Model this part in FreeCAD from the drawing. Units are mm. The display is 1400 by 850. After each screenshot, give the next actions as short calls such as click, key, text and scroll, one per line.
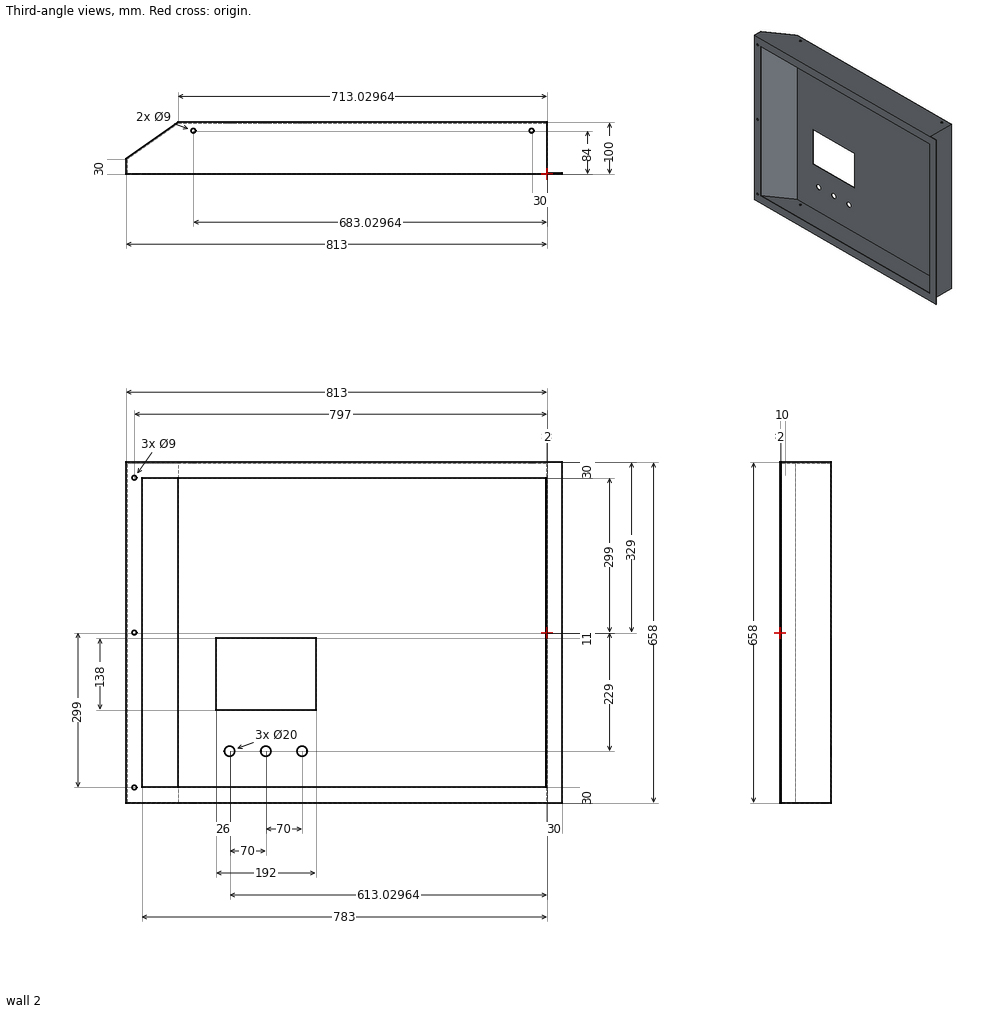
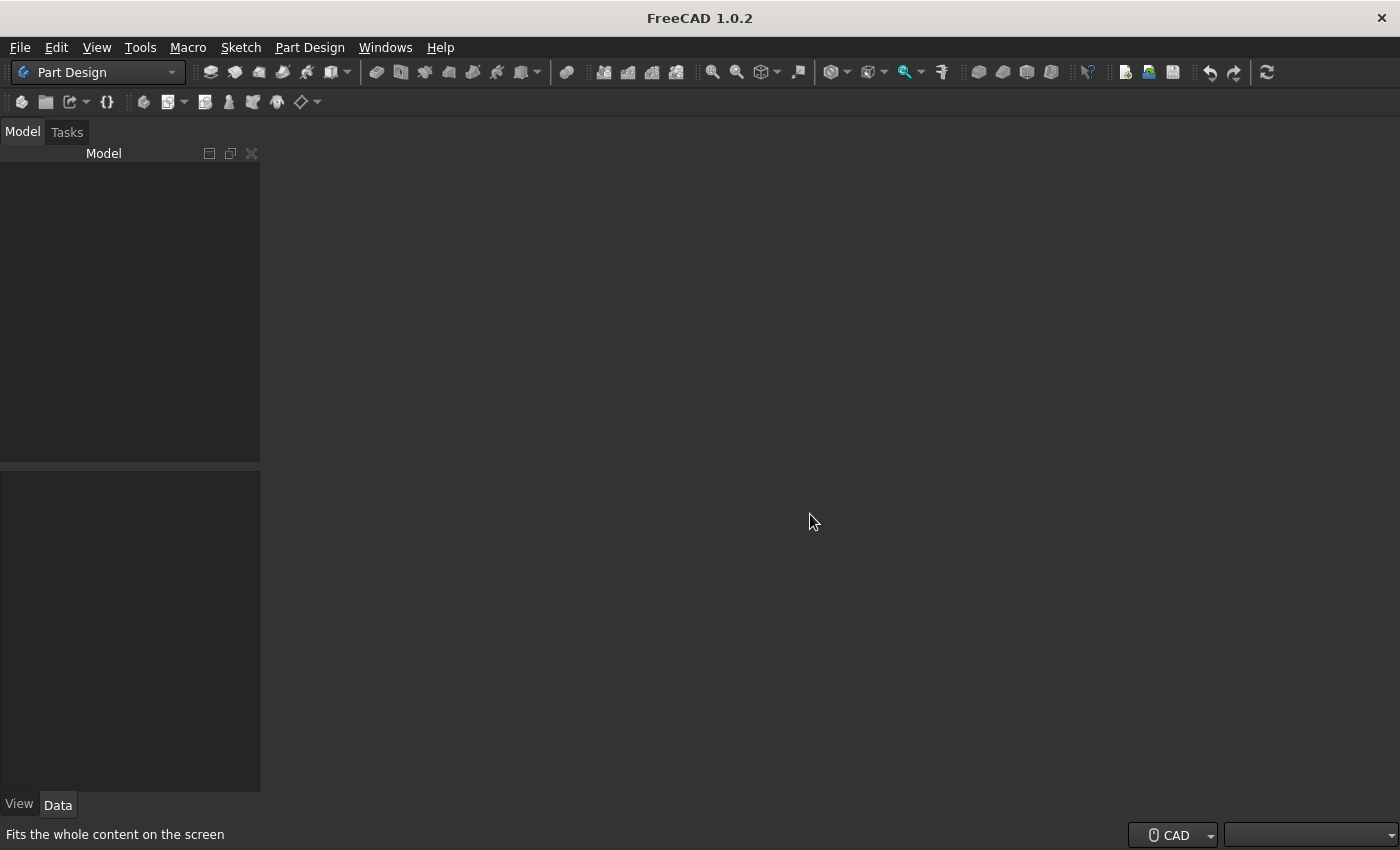
click(1126, 72)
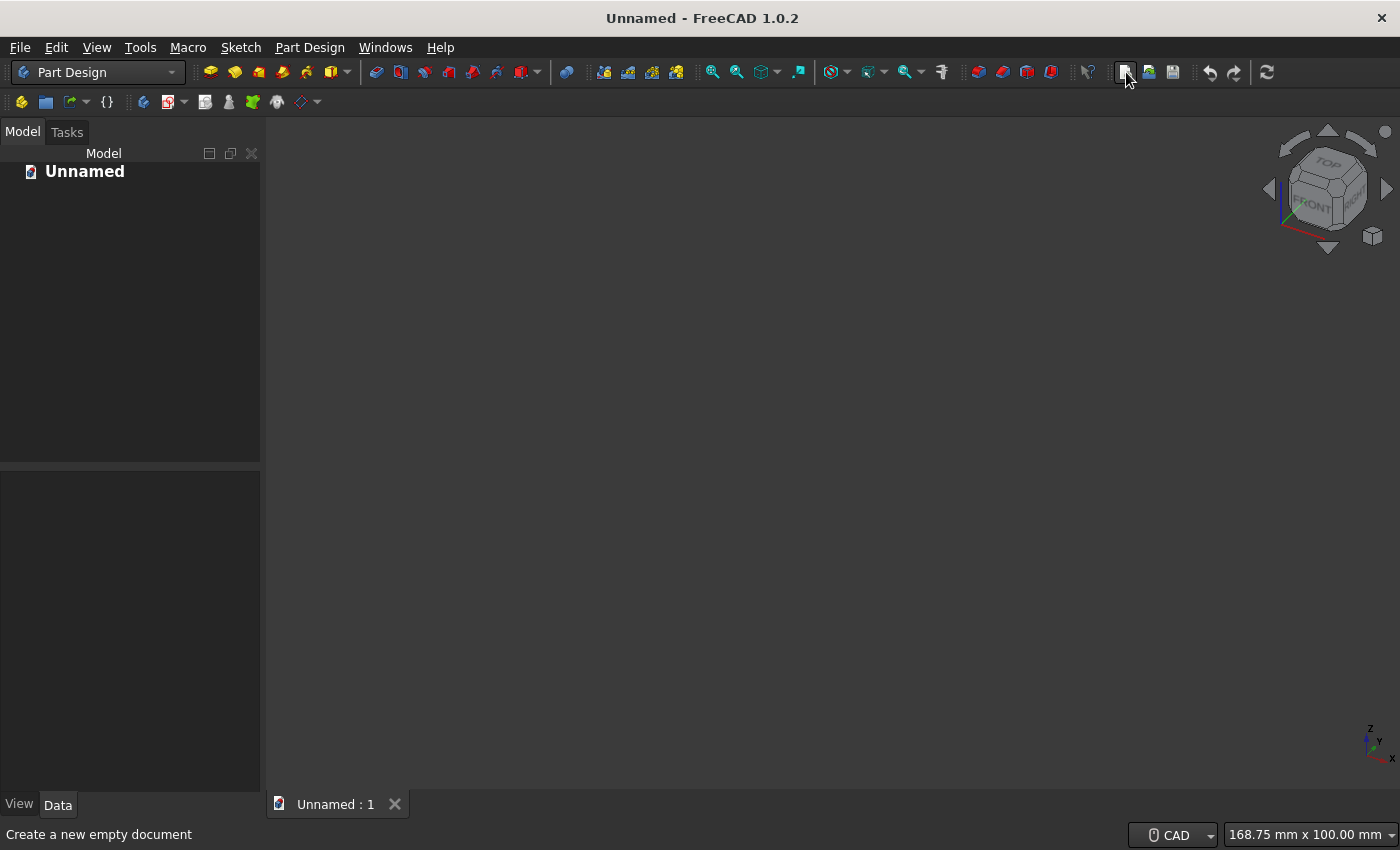
click(168, 102)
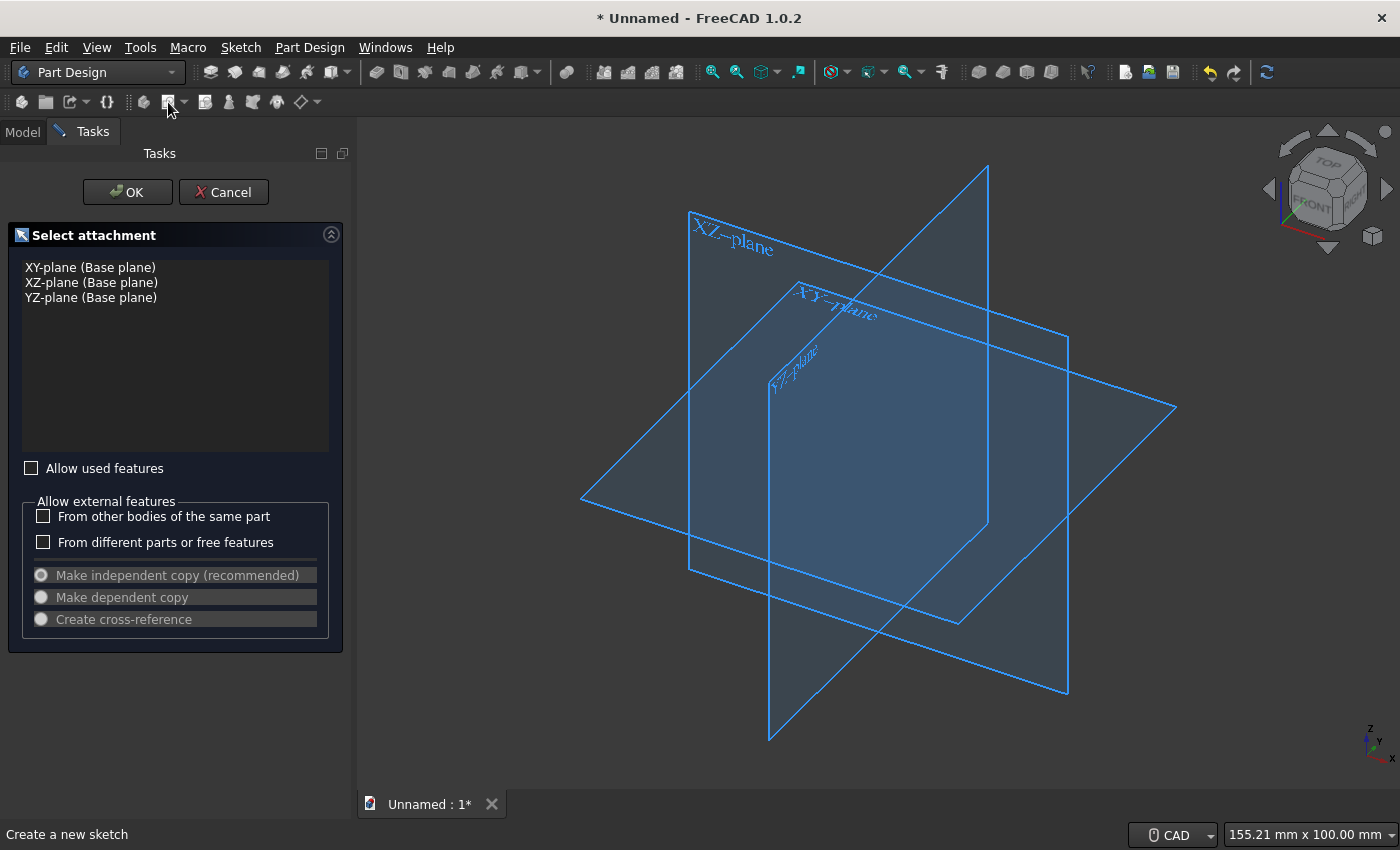
click(82, 268)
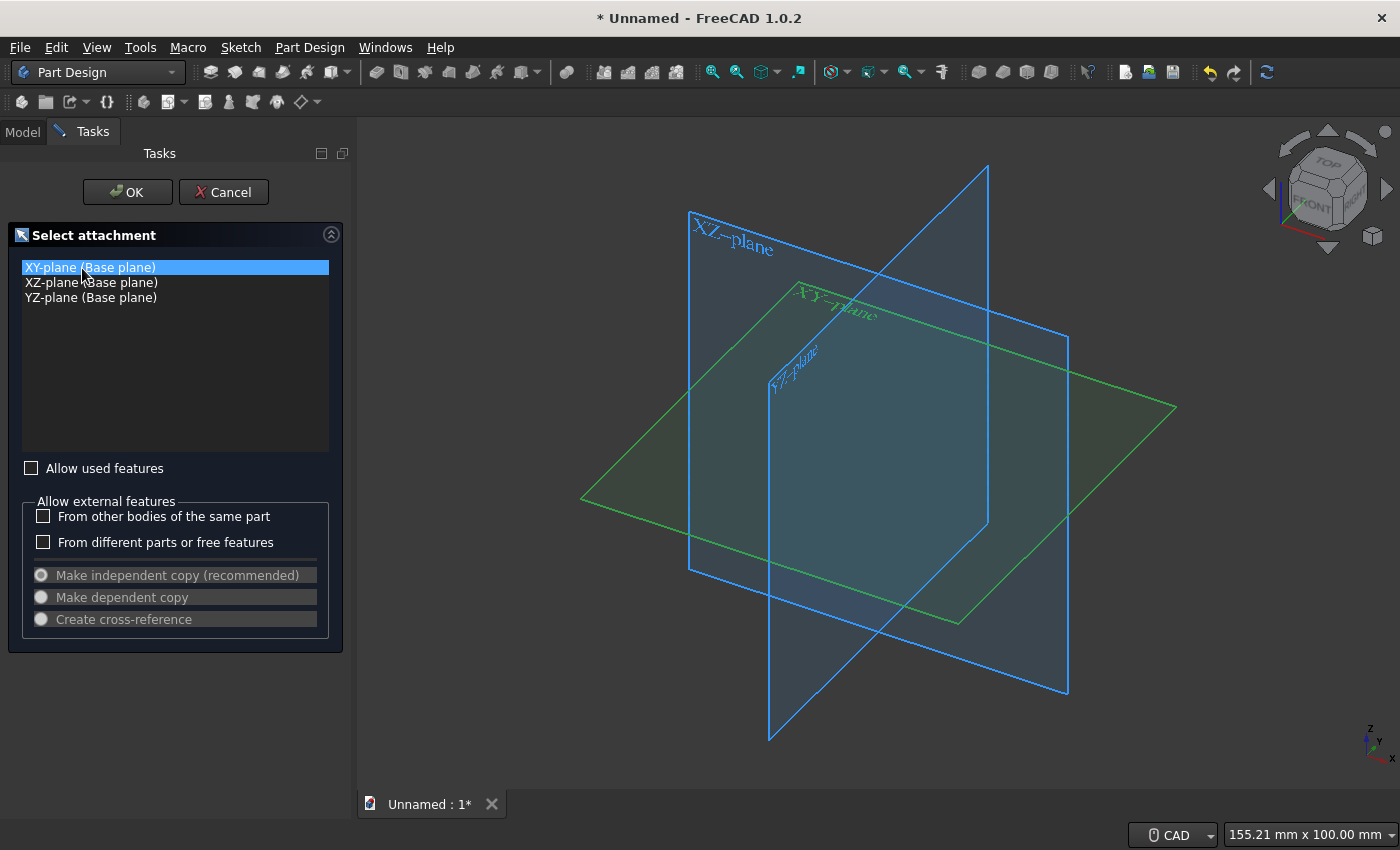
click(128, 192)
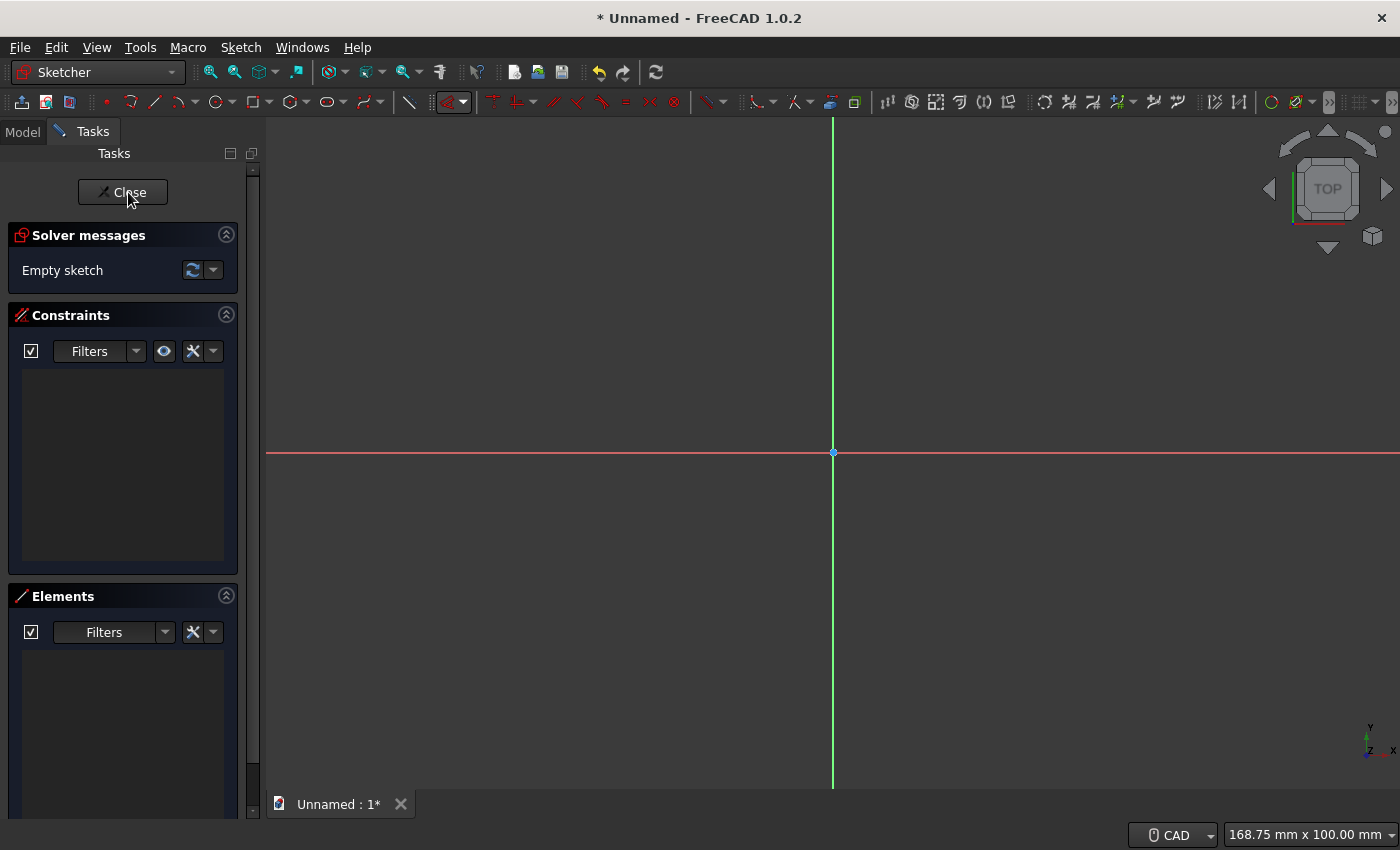
scroll(1096, 495, down, 11)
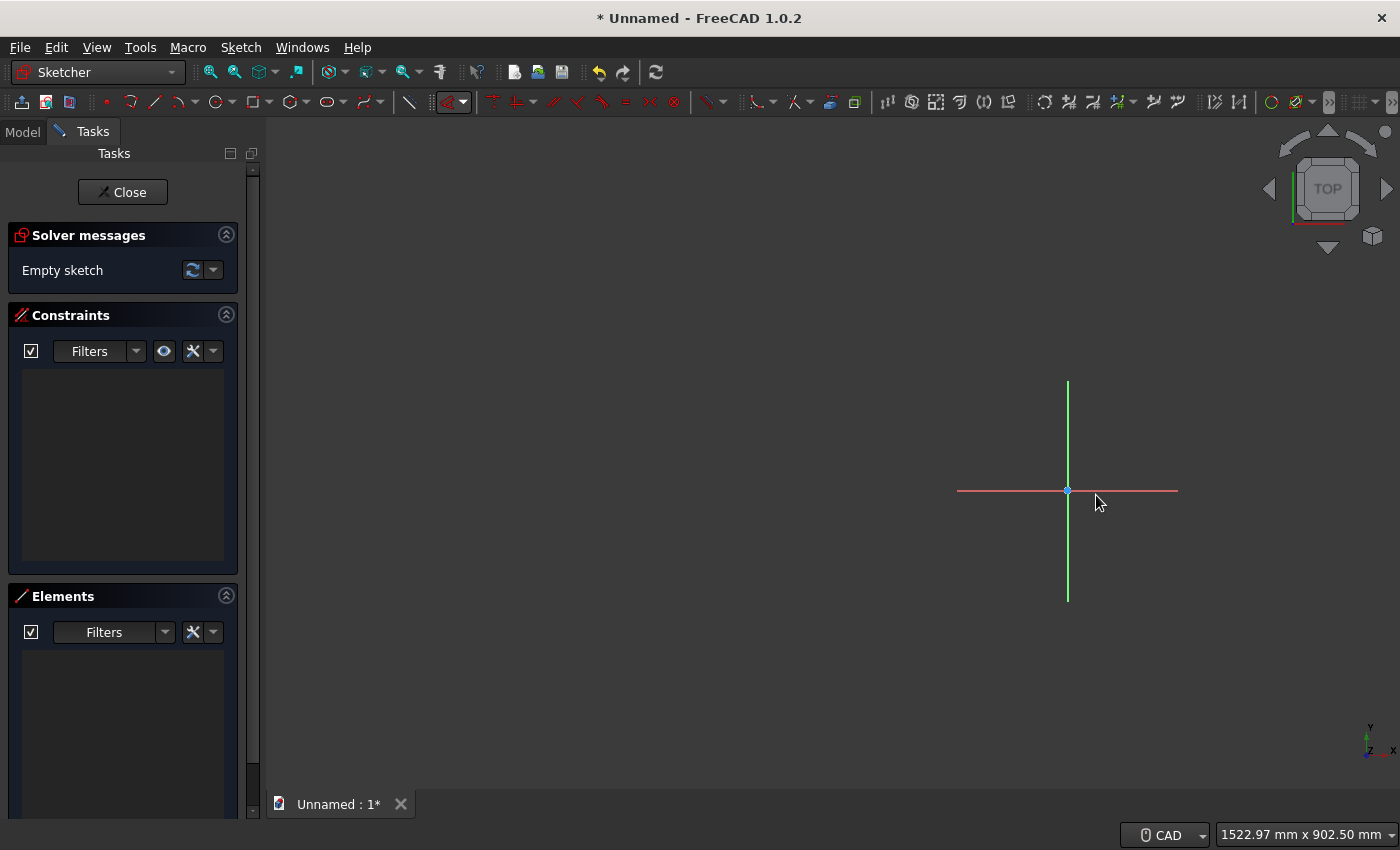
click(132, 102)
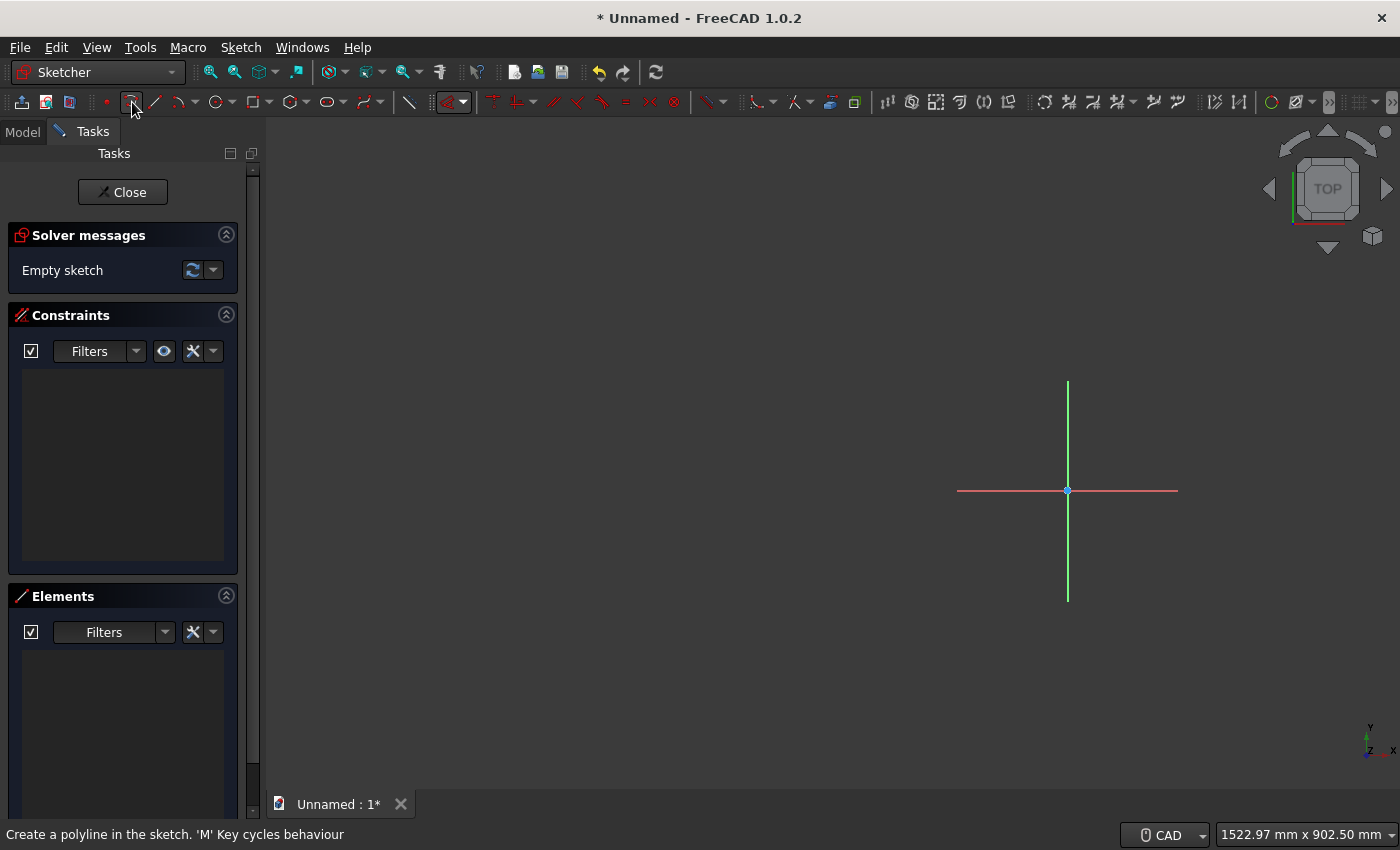
click(1068, 491)
click(1059, 416)
click(537, 416)
click(462, 469)
click(462, 482)
click(1068, 491)
key(Escape)
key(Escape)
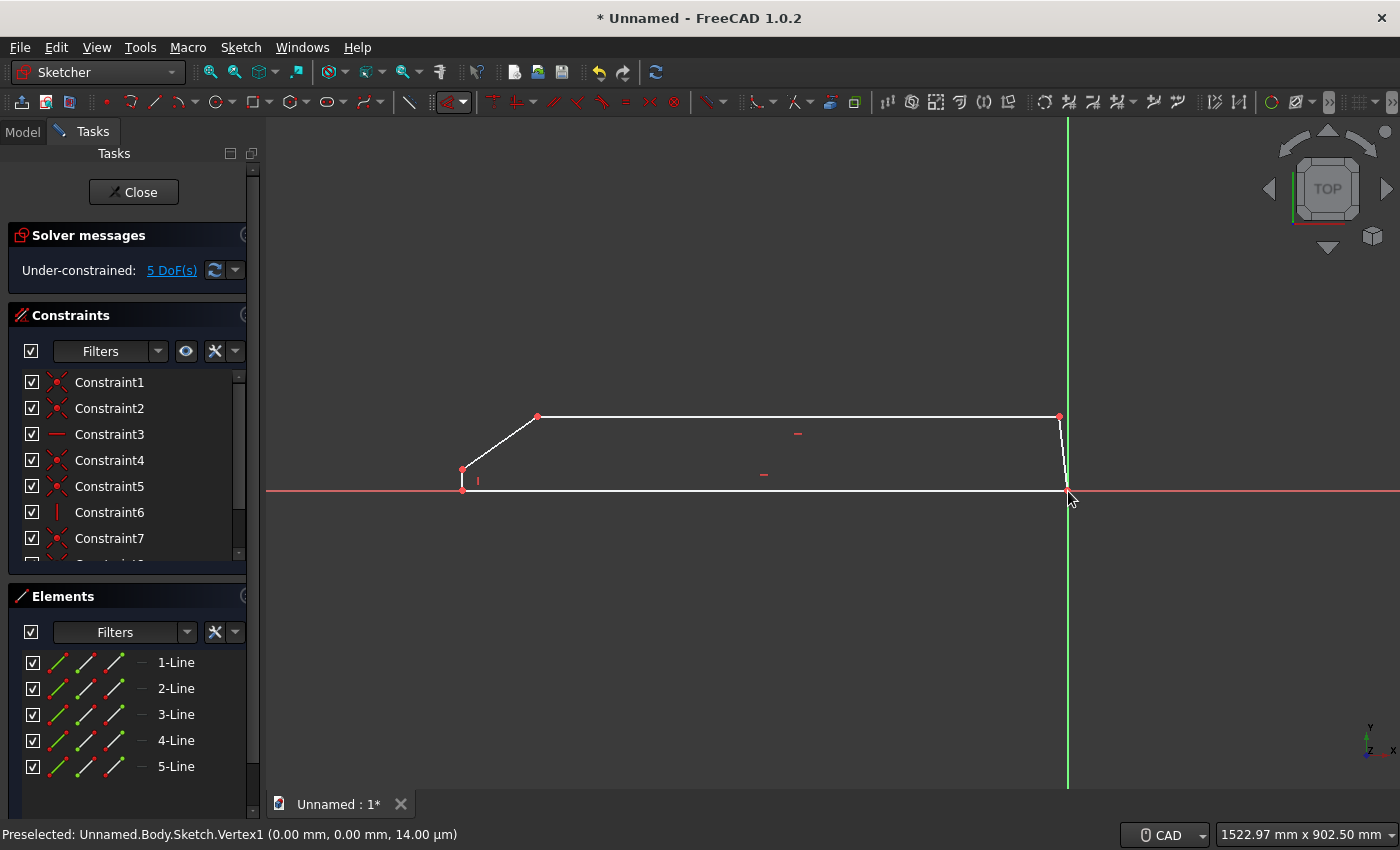
click(1065, 469)